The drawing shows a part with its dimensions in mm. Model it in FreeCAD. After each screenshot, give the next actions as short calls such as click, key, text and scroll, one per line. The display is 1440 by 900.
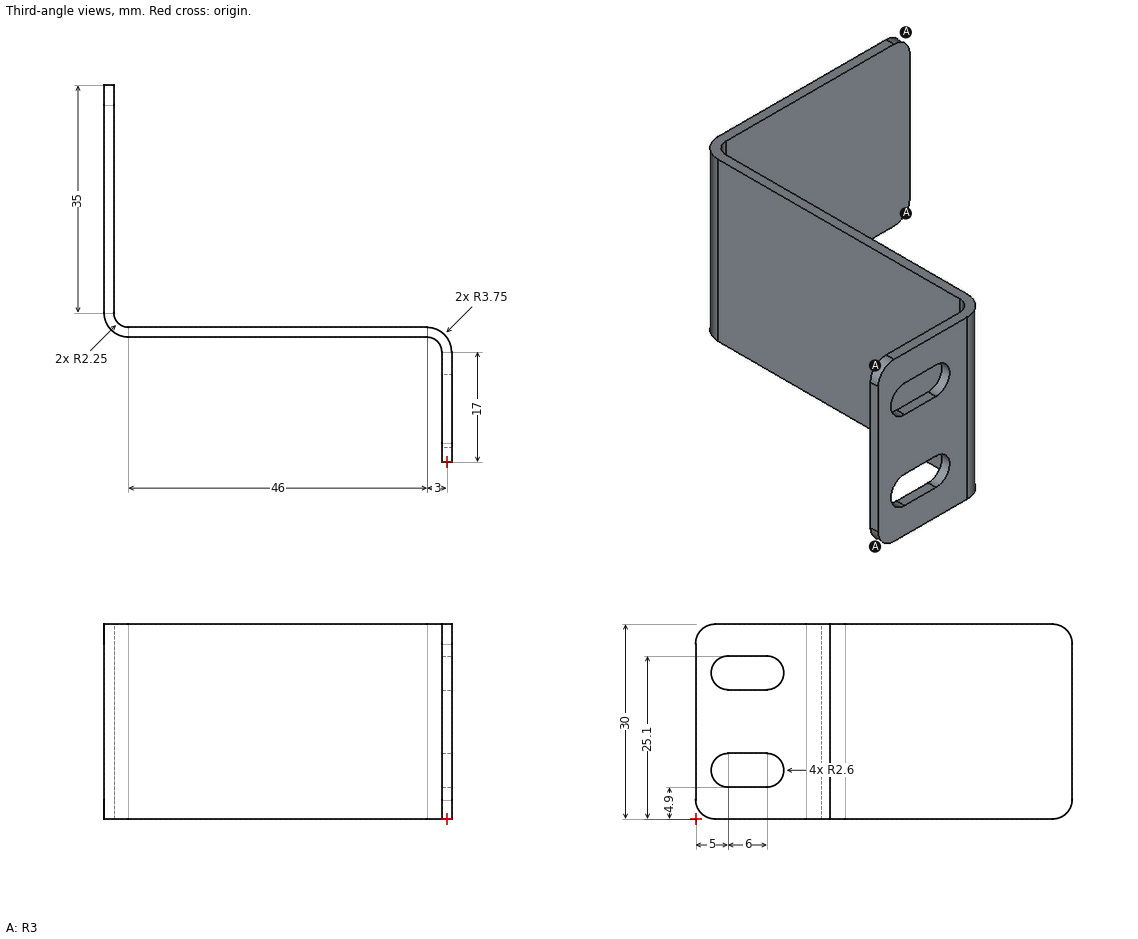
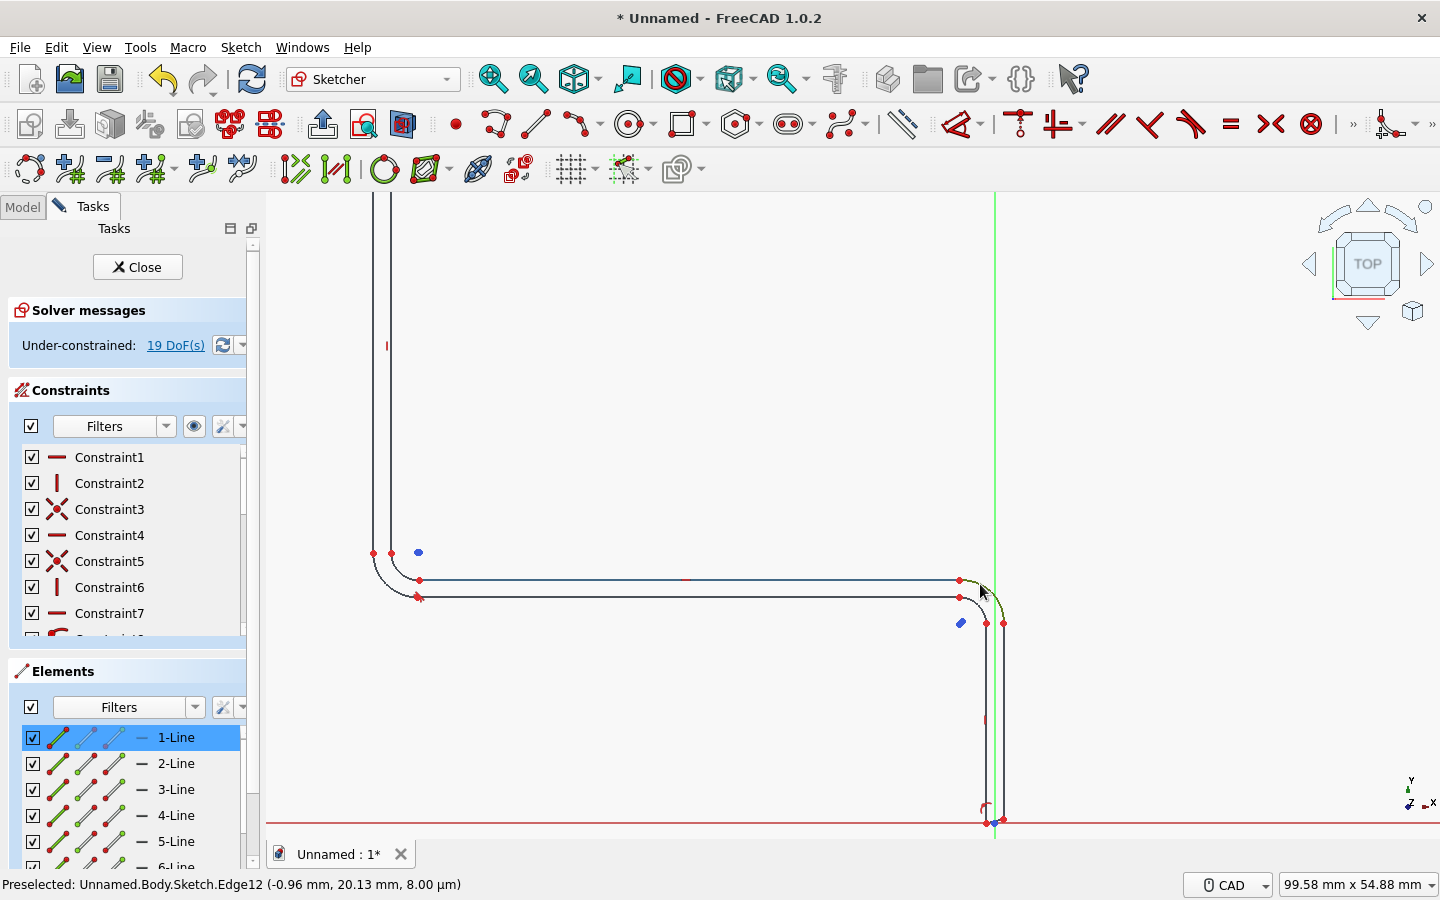
key(t)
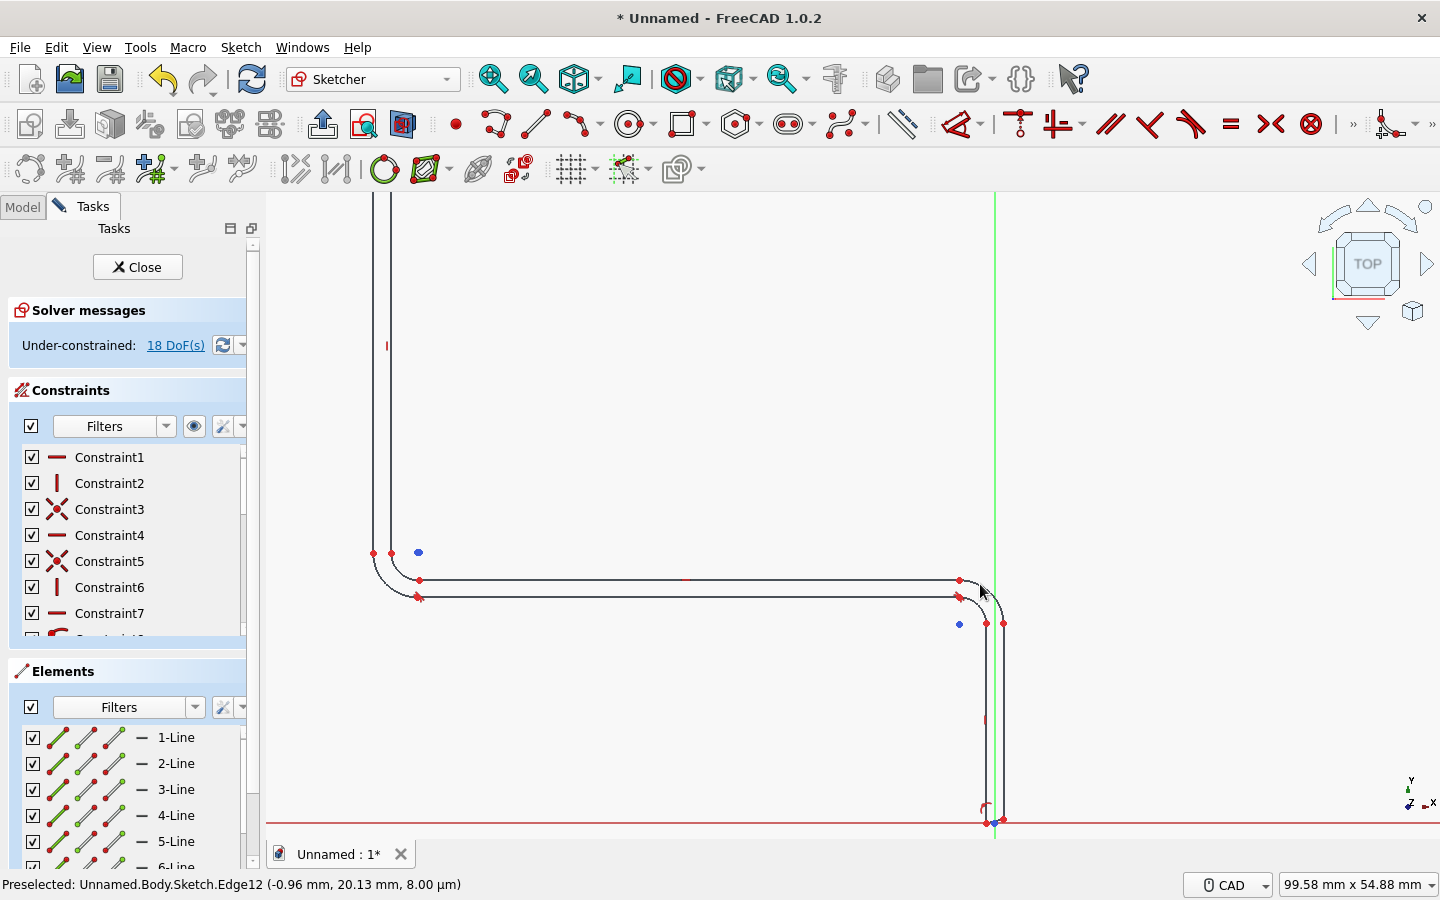
click(391, 430)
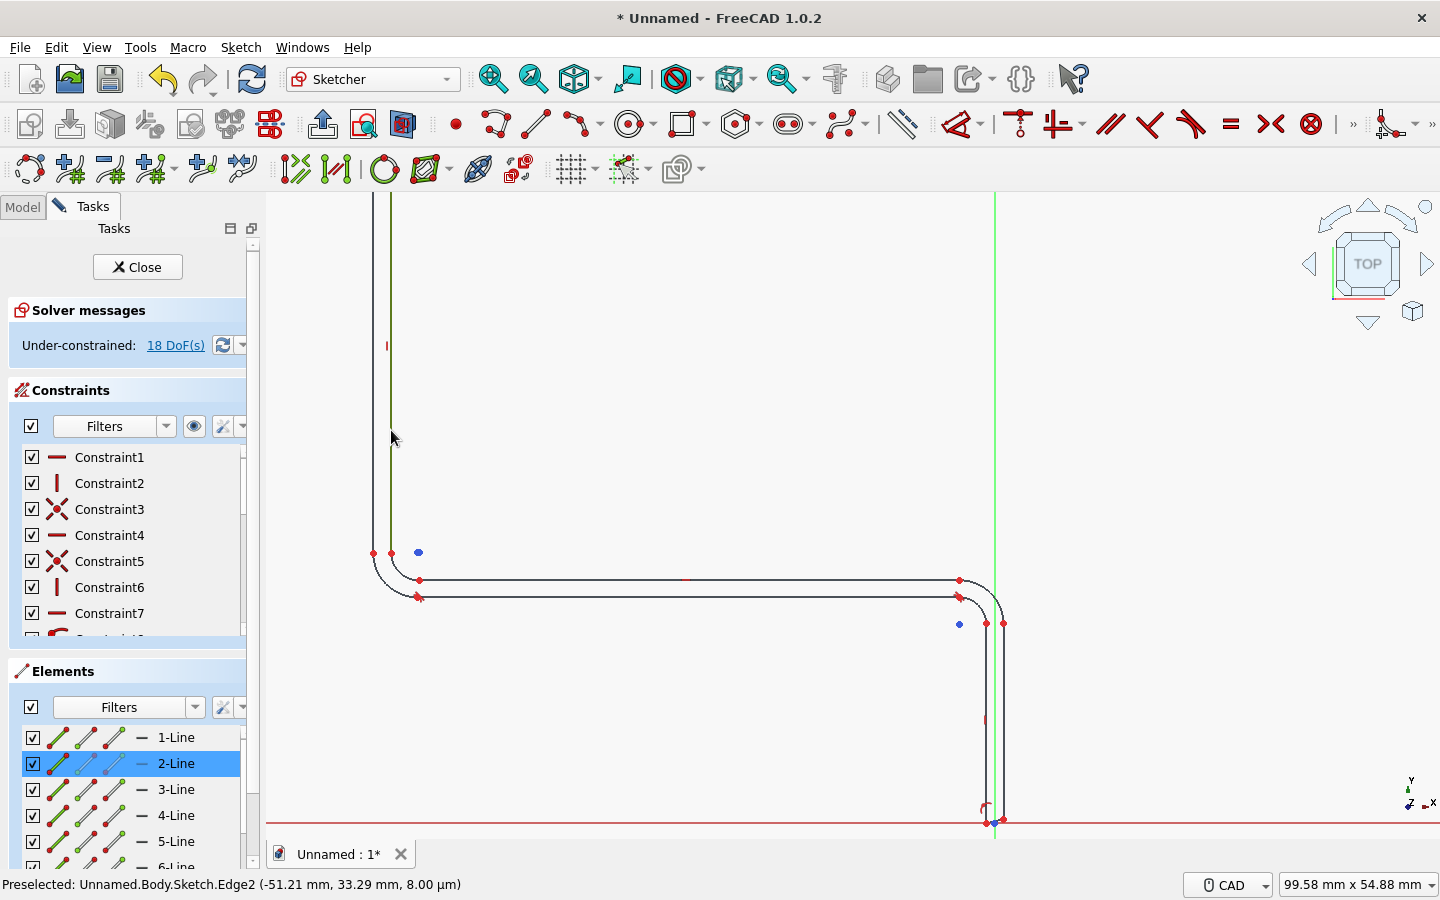
click(394, 566)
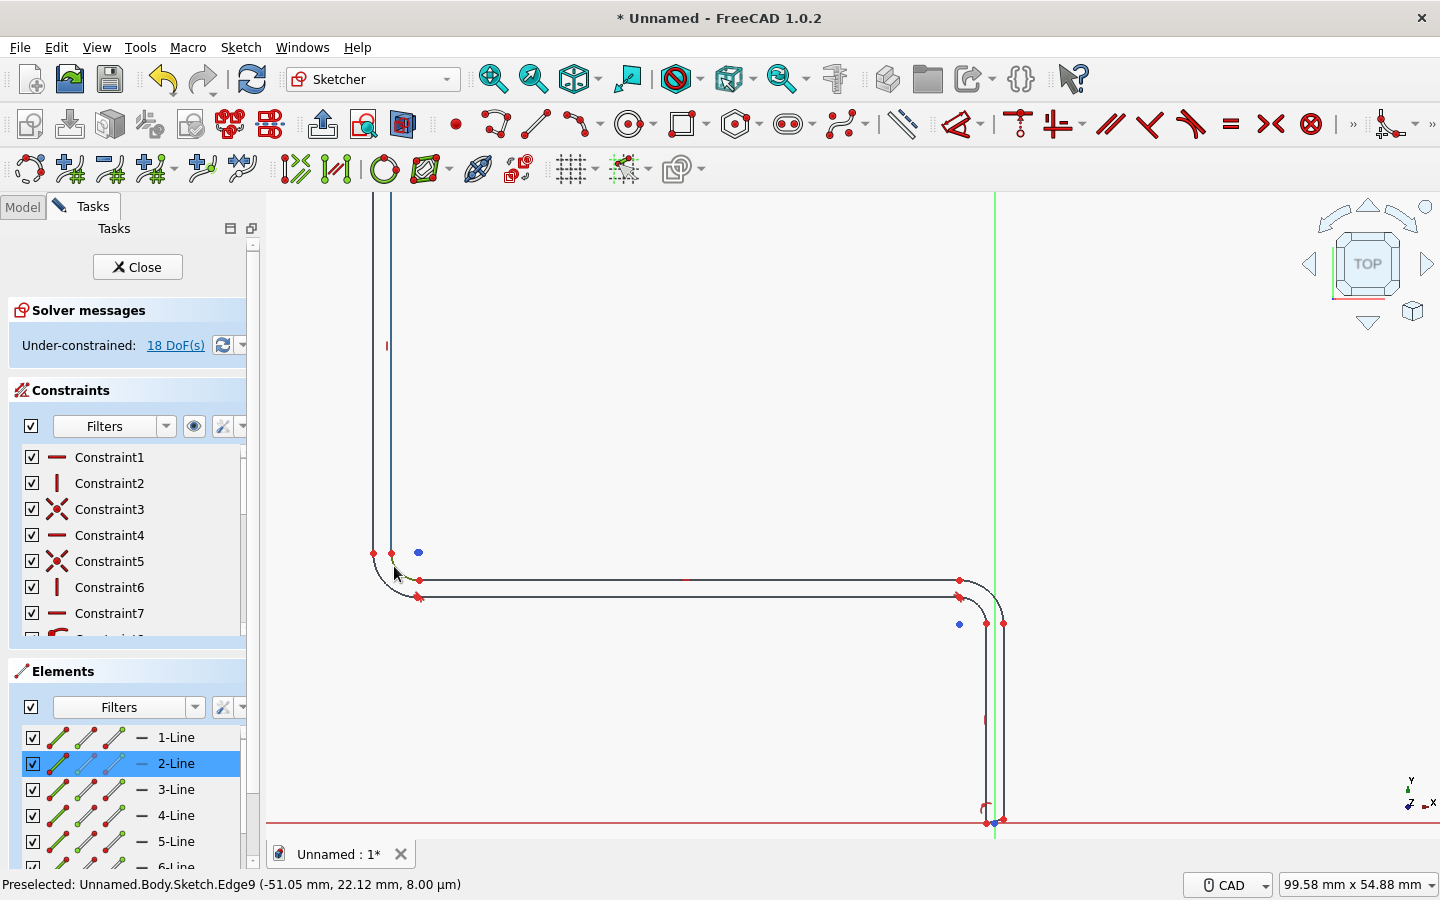
key(t)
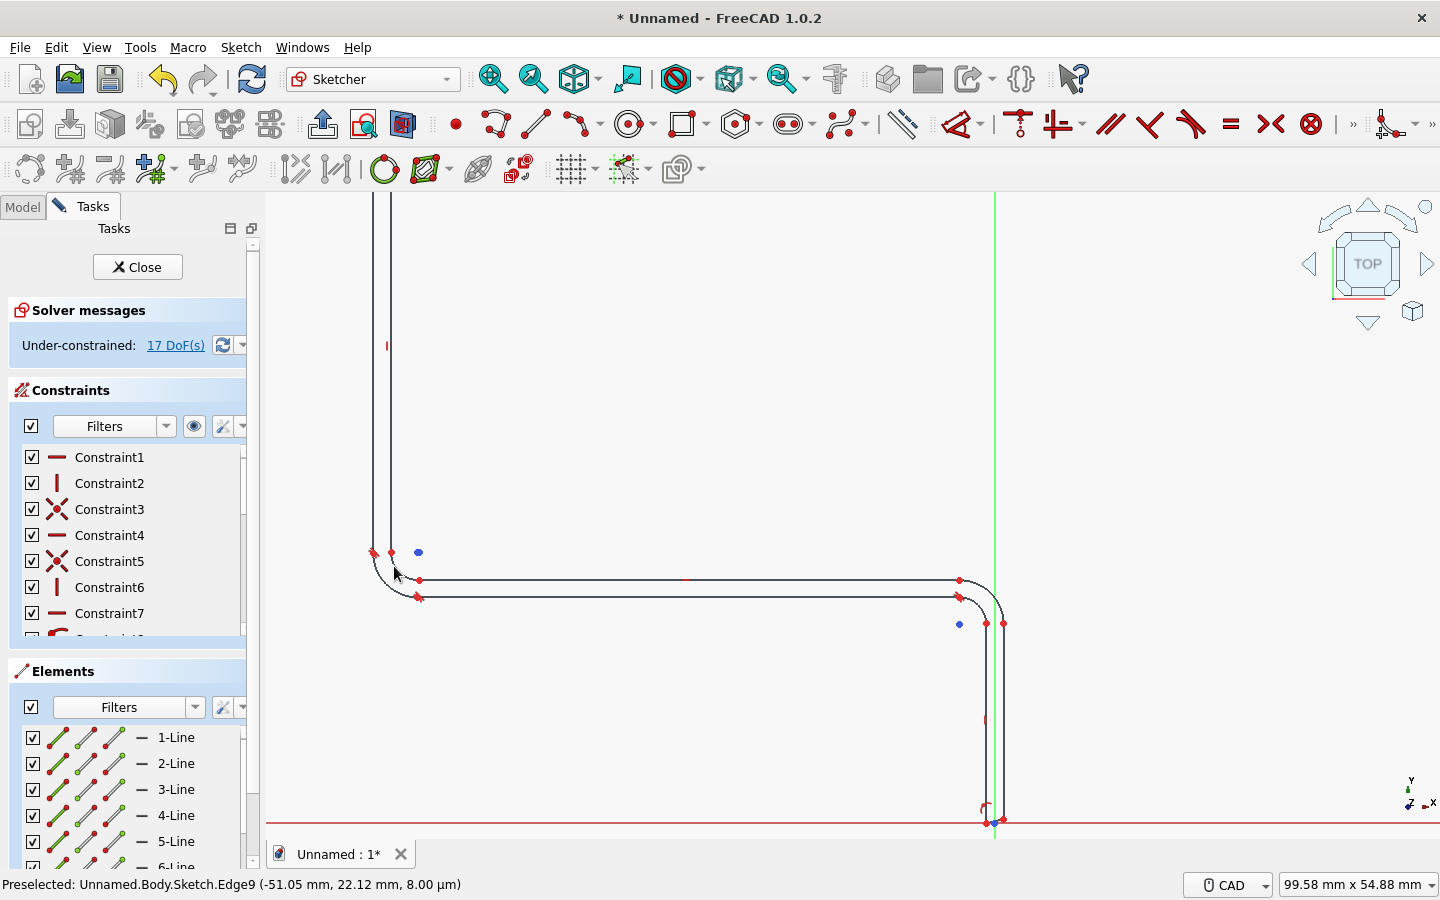
click(373, 265)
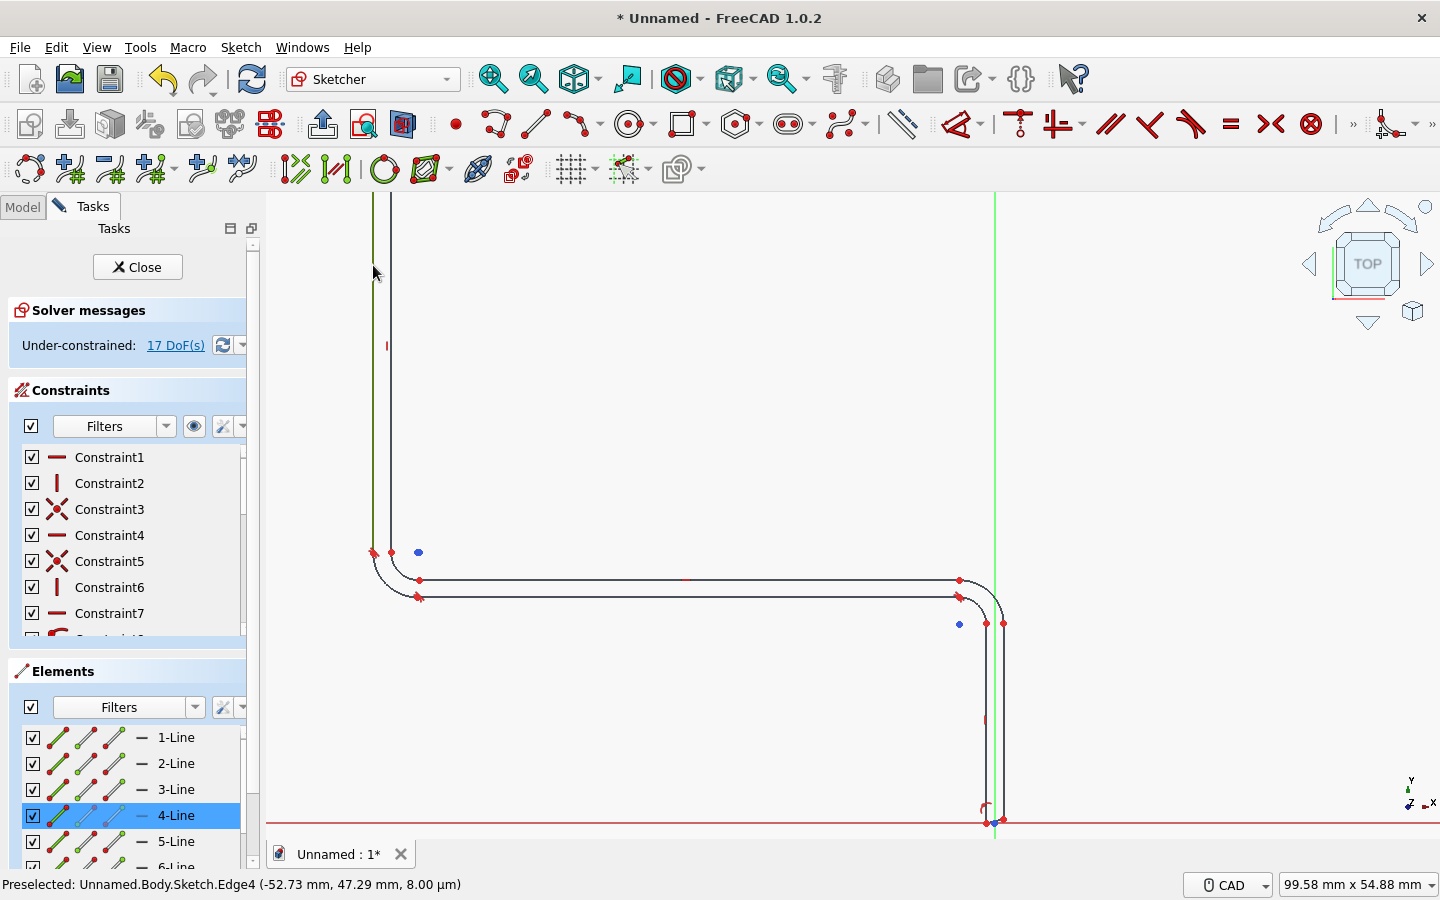
click(378, 573)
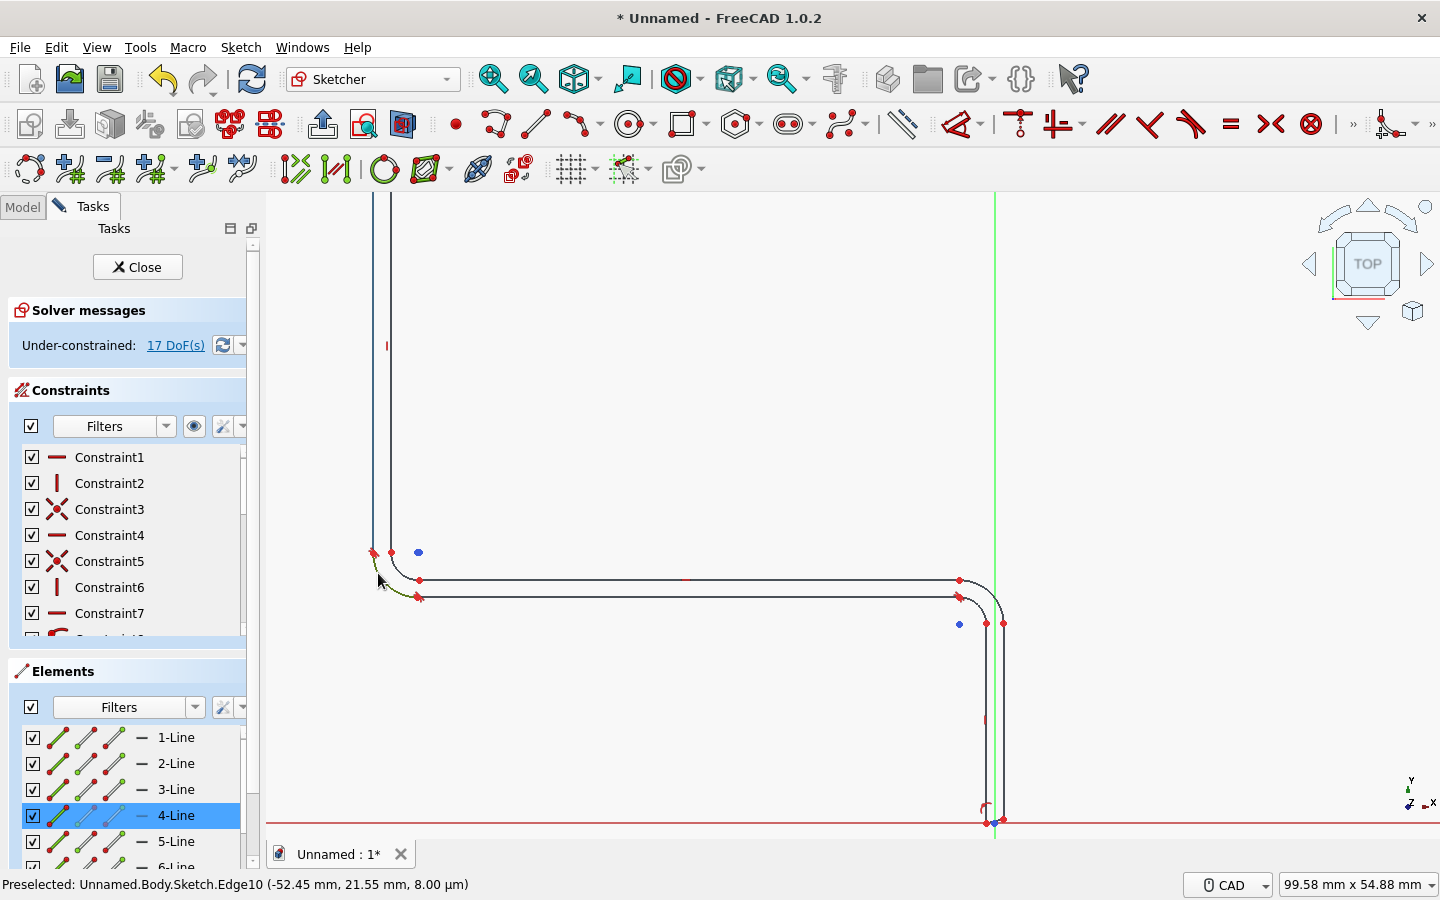
key(t)